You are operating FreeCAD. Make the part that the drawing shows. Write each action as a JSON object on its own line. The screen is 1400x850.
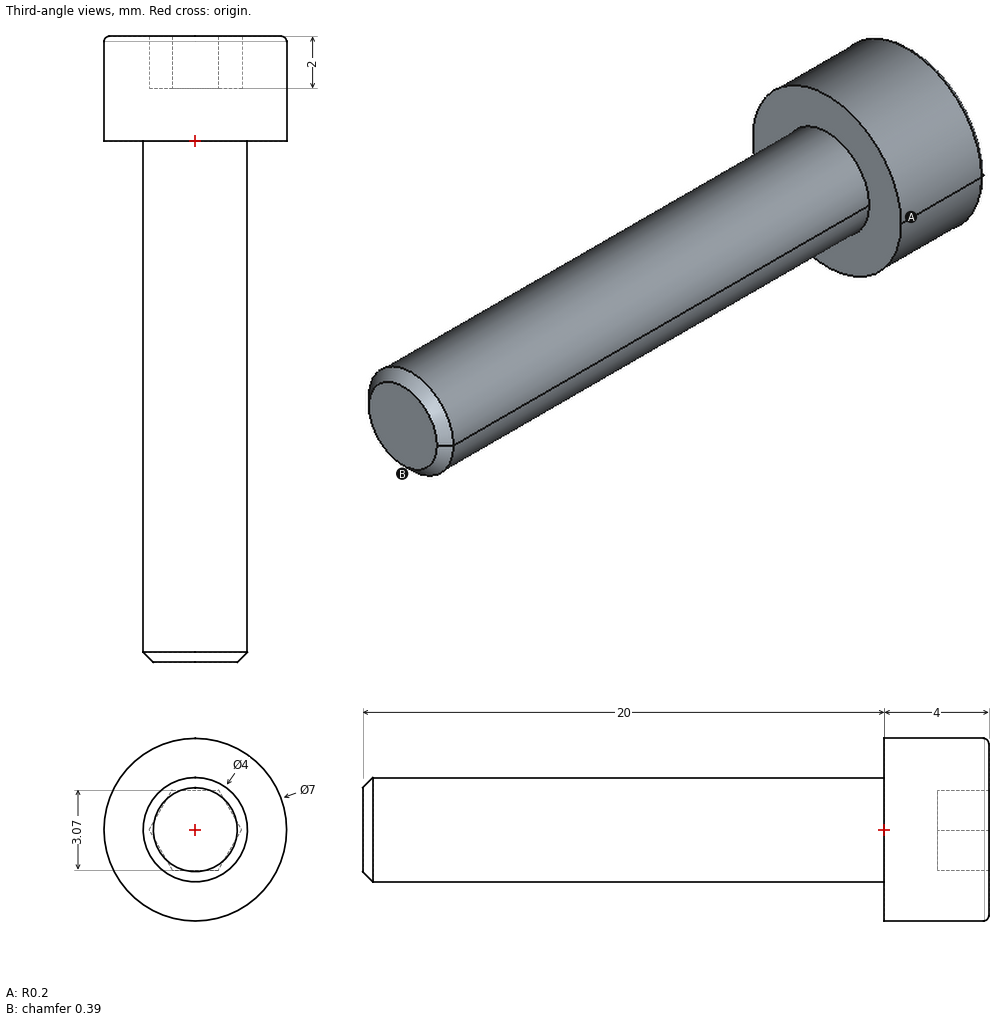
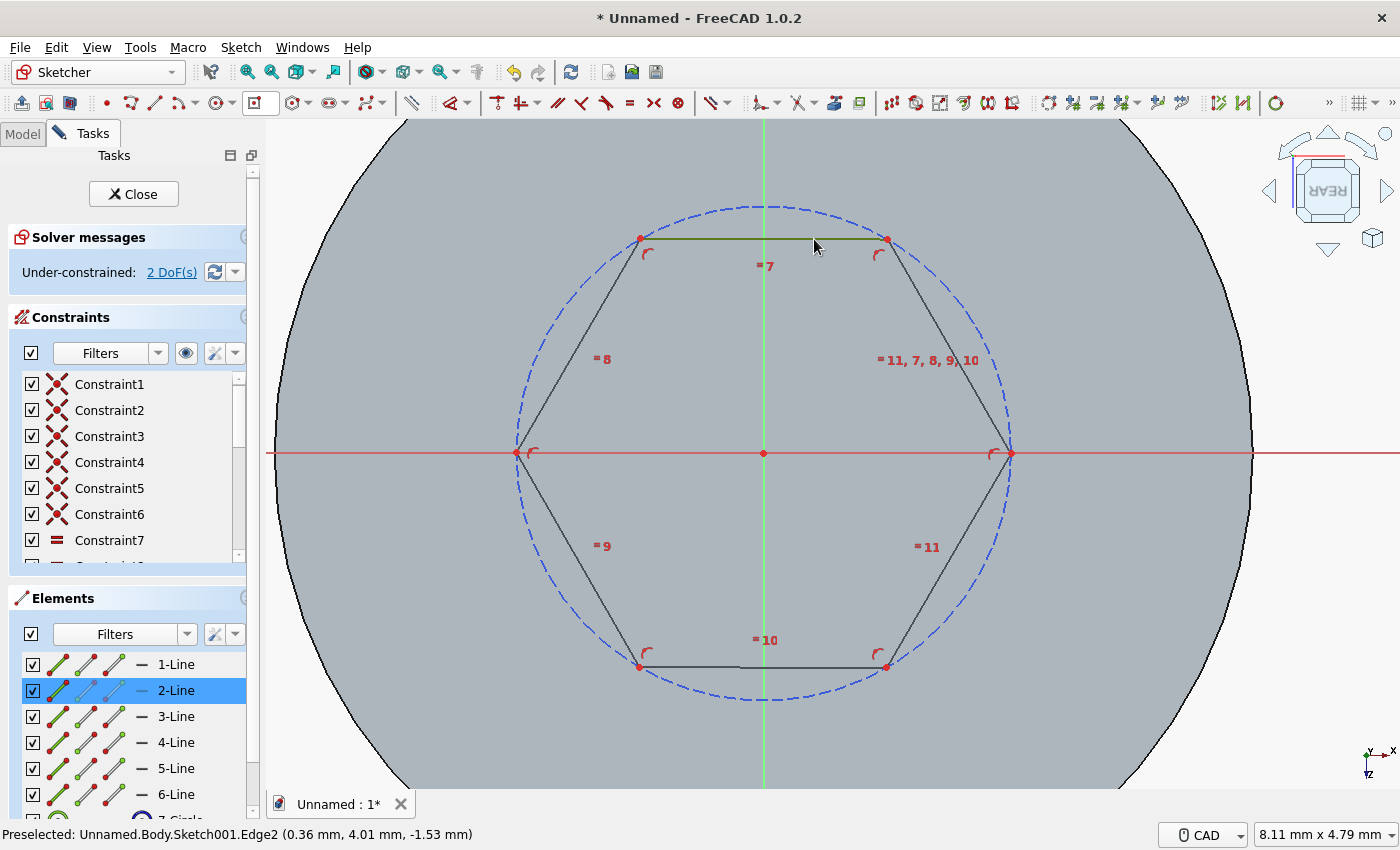
{"action": "key", "text": "h"}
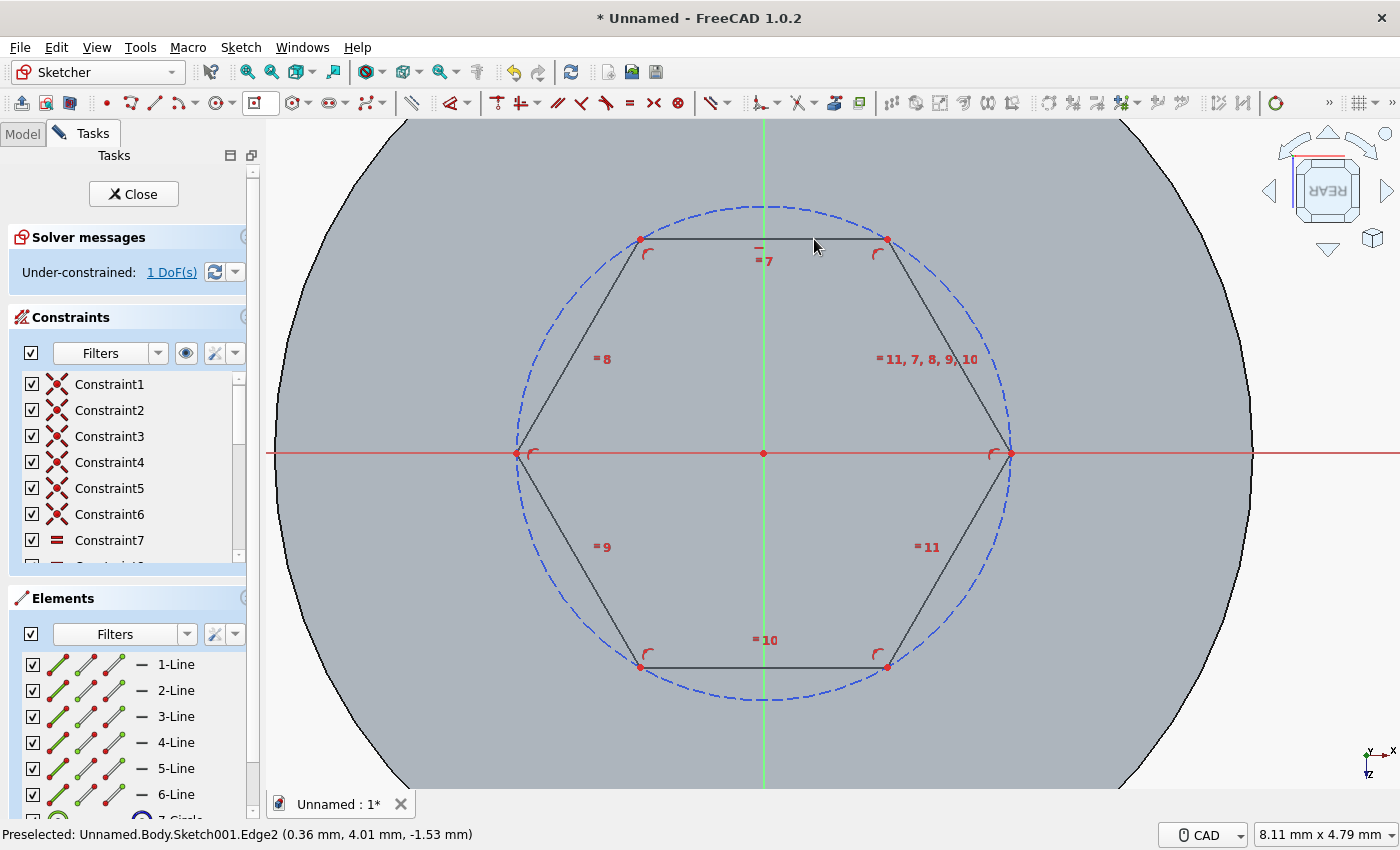
{"action": "key", "text": "d"}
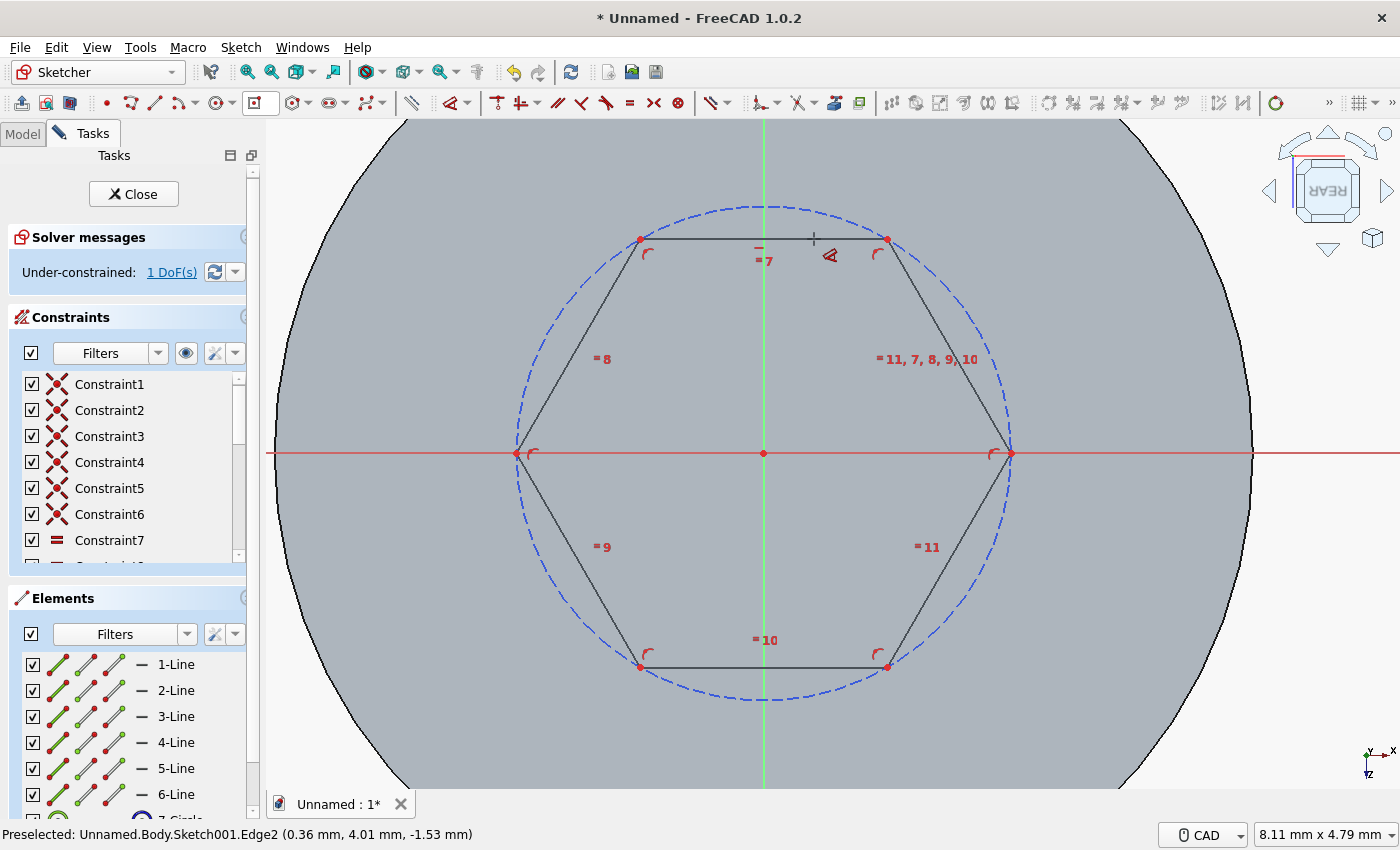
{"action": "left_click", "coordinate": [640, 668]}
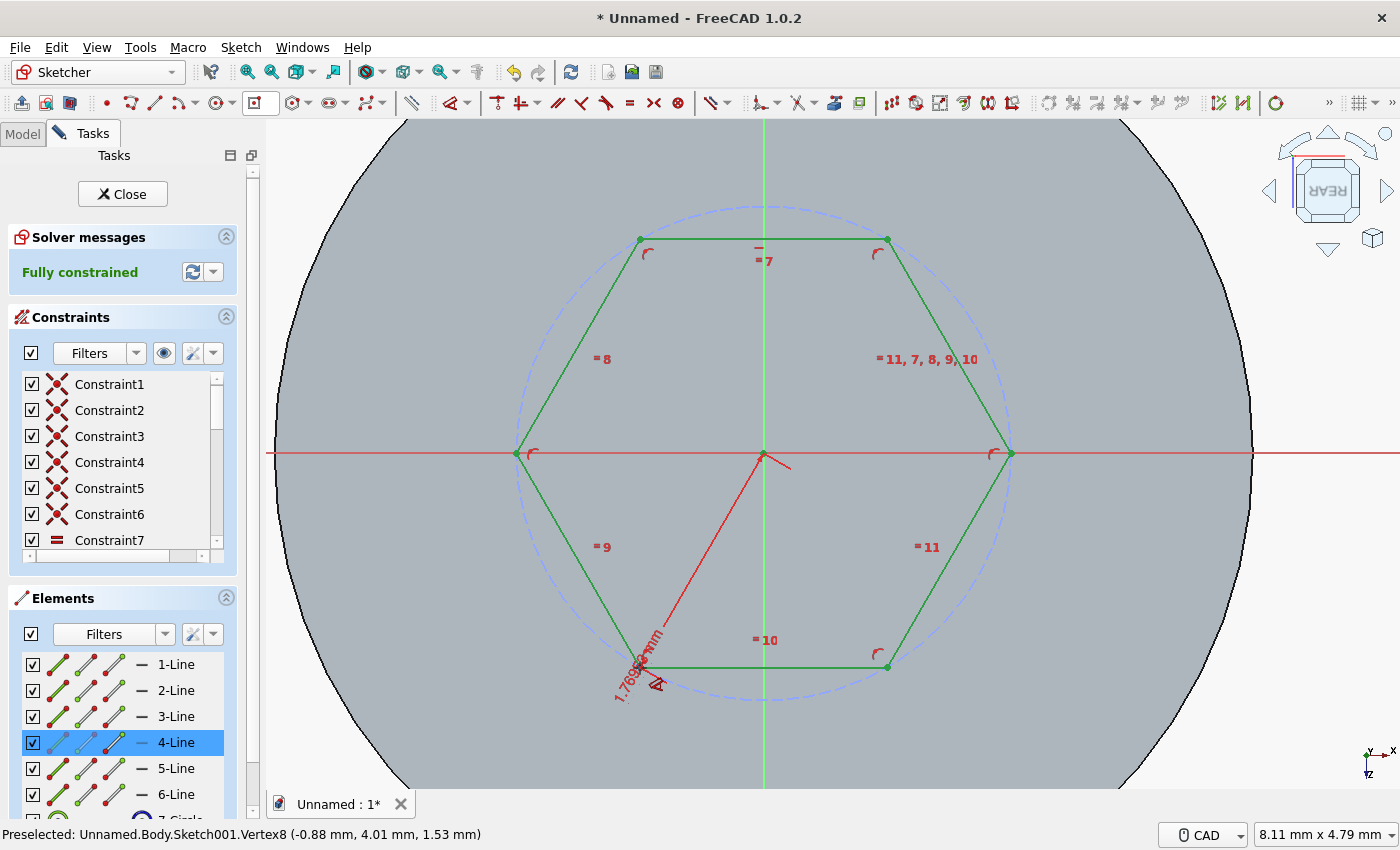
{"action": "left_click", "coordinate": [887, 239]}
{"action": "left_click", "coordinate": [606, 355]}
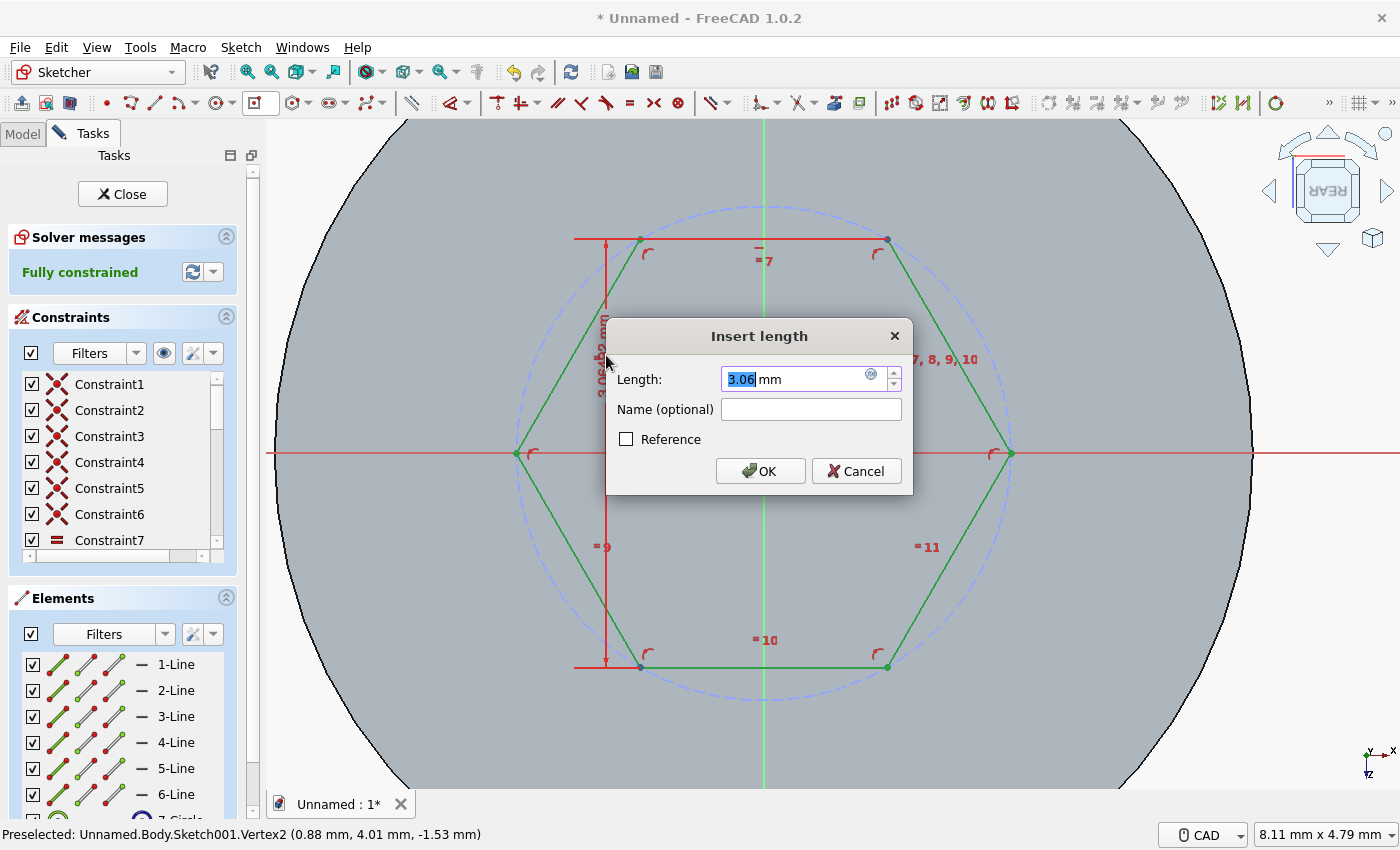
{"action": "type", "text": "3.07"}
{"action": "key", "text": "Return"}
{"action": "key", "text": "Escape"}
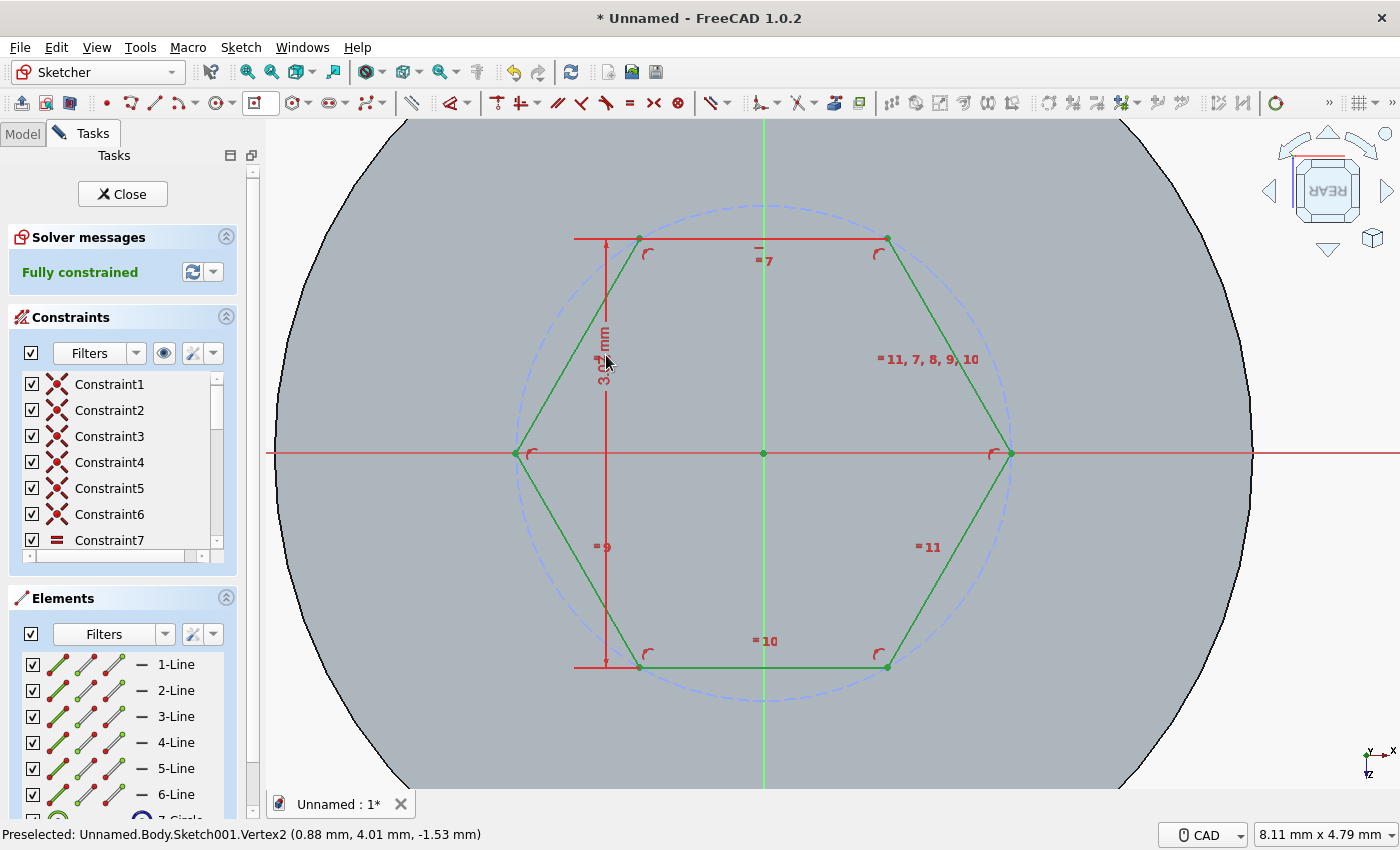
{"action": "left_click", "coordinate": [123, 194]}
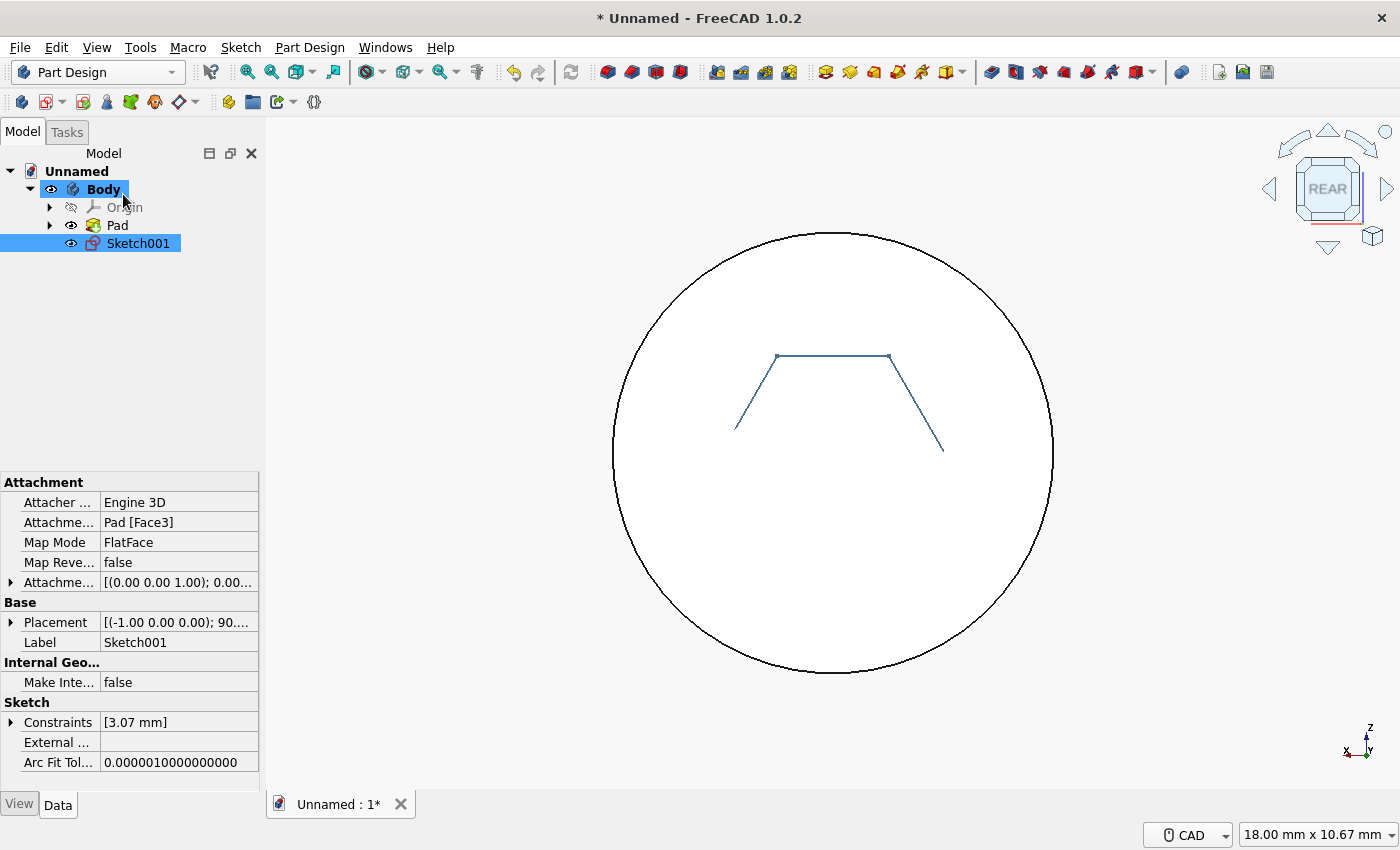
{"action": "left_click", "coordinate": [992, 72]}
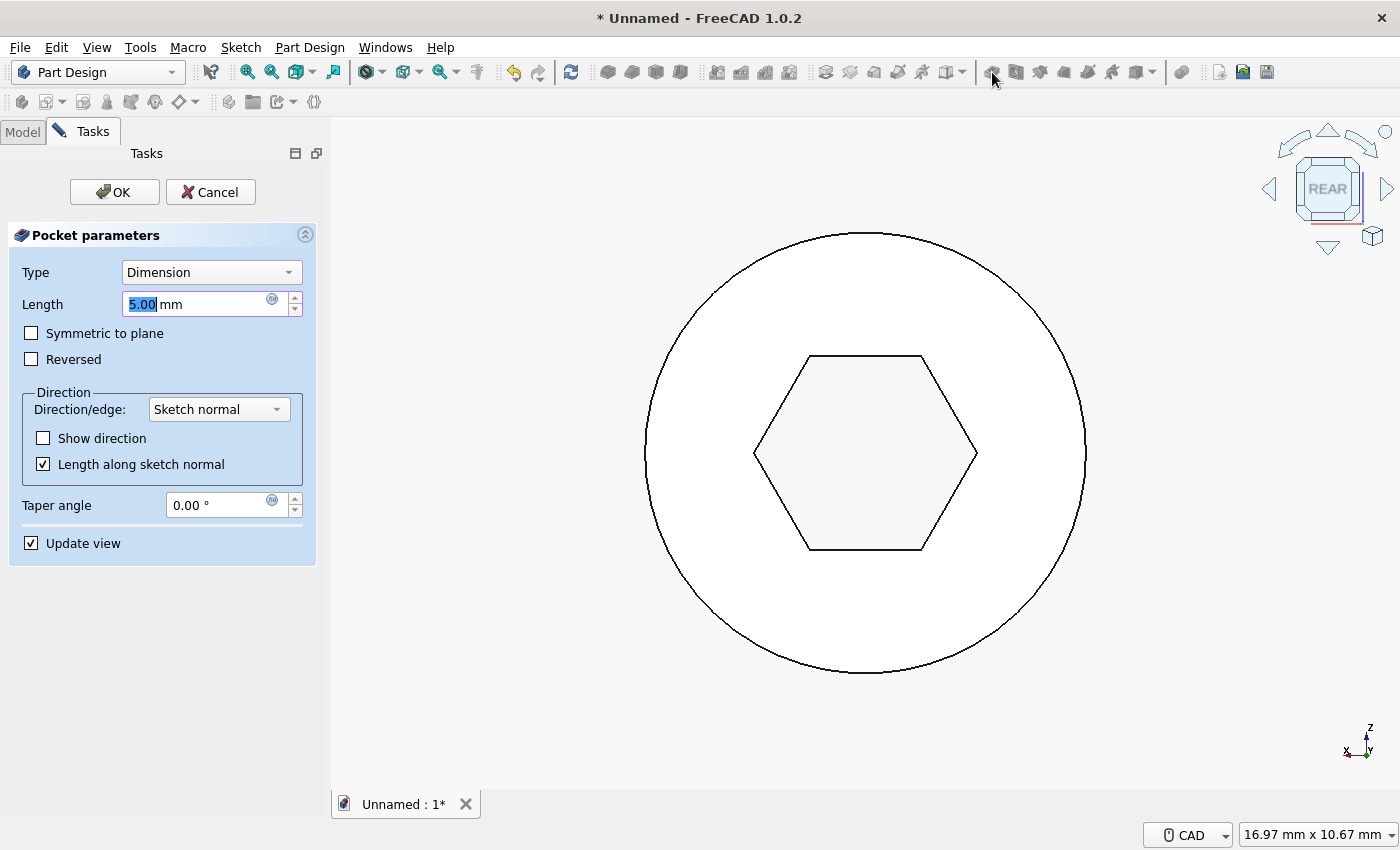
{"action": "type", "text": "2"}
{"action": "key", "text": "Tab"}